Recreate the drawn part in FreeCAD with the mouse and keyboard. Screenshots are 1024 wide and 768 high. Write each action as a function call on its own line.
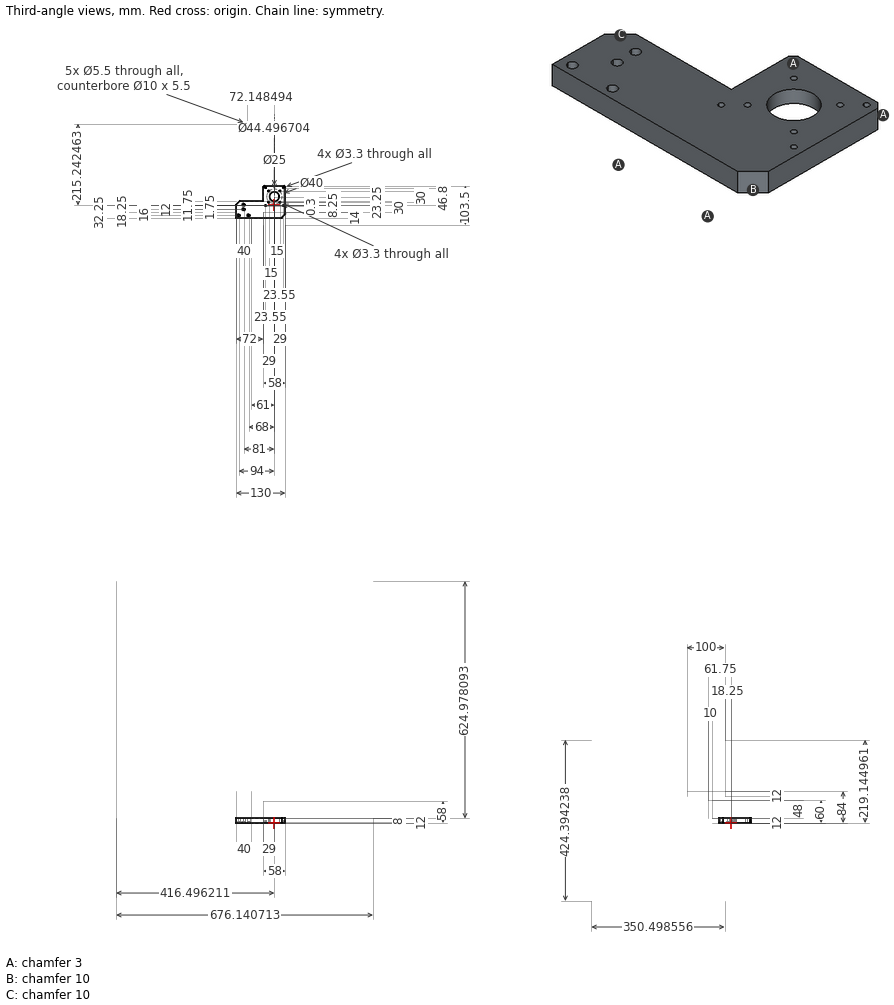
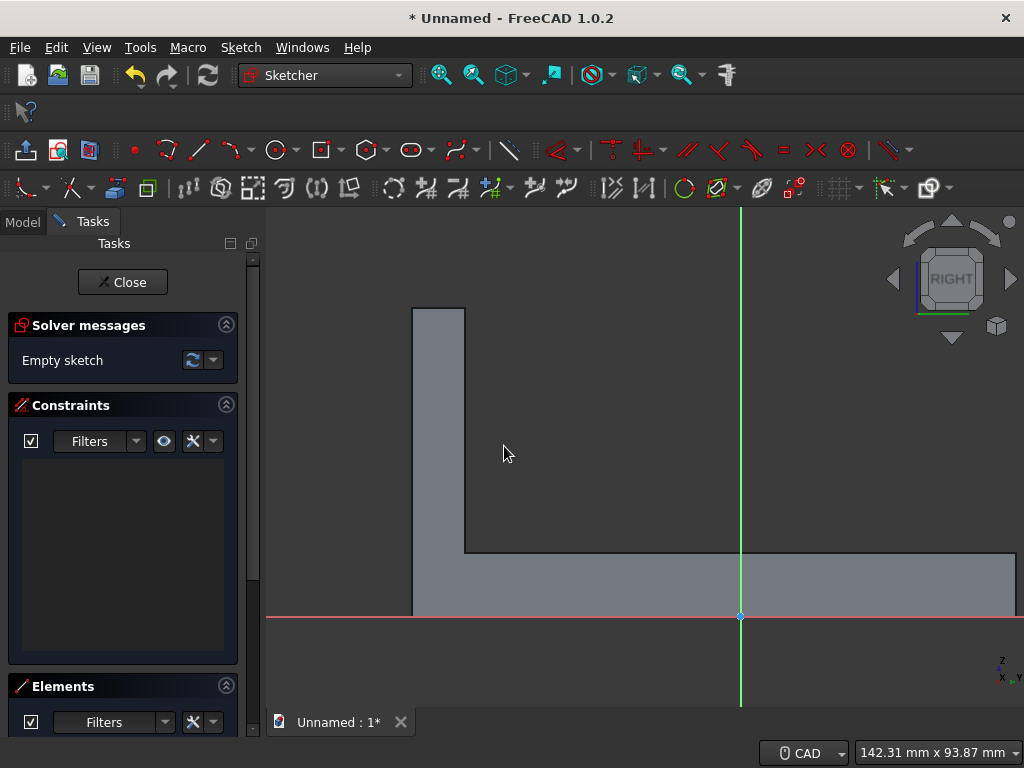
click(344, 150)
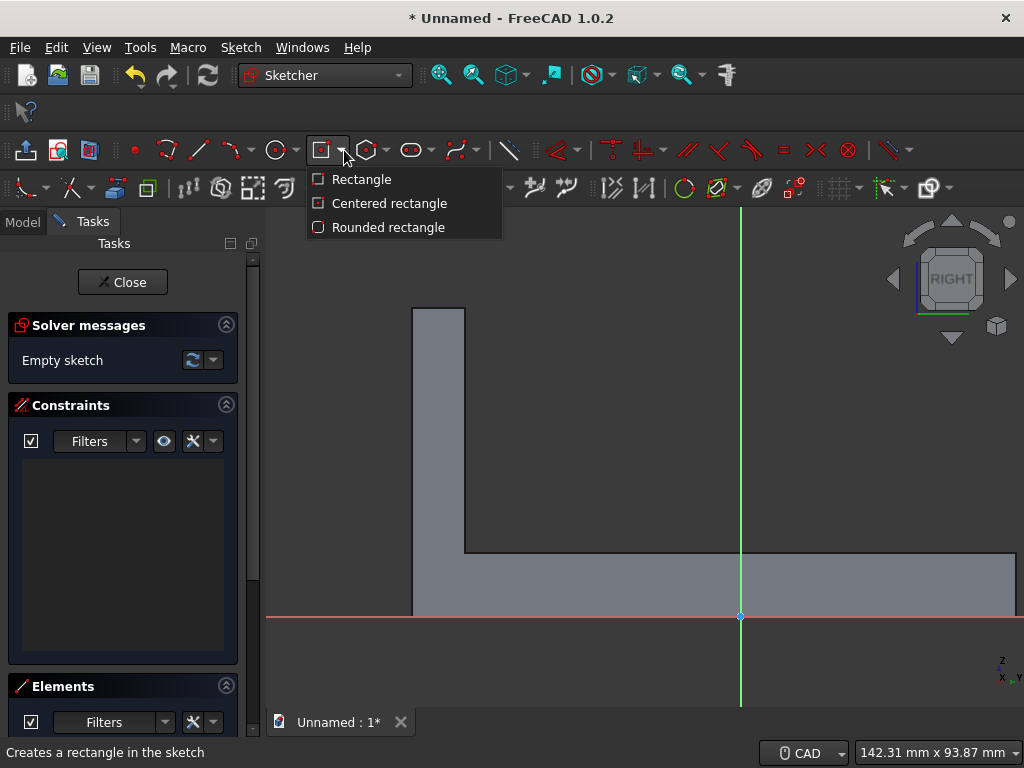
click(404, 179)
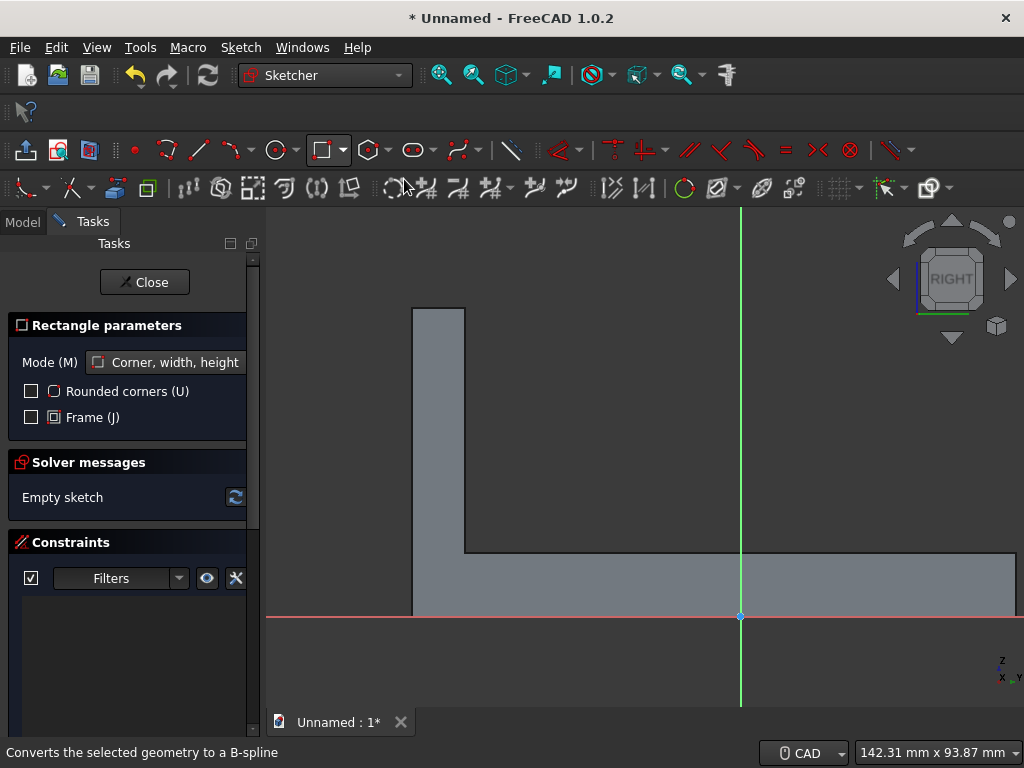
click(412, 297)
move(465, 553)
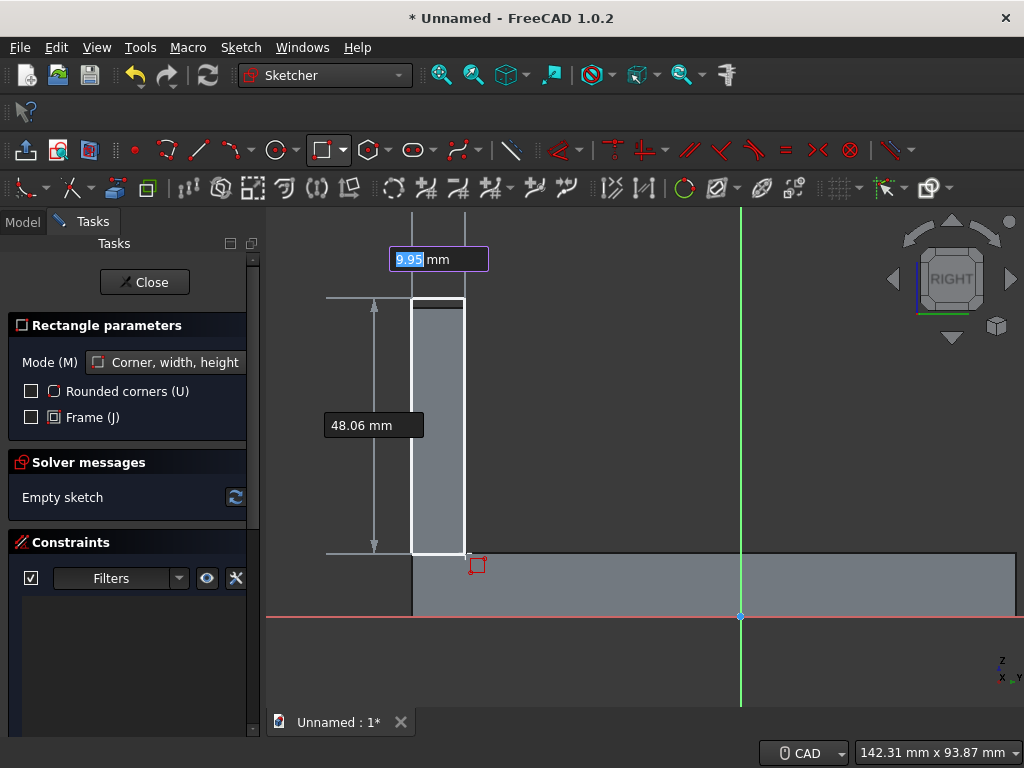
text(10)
key(Tab)
text(48)
key(Return)
key(Escape)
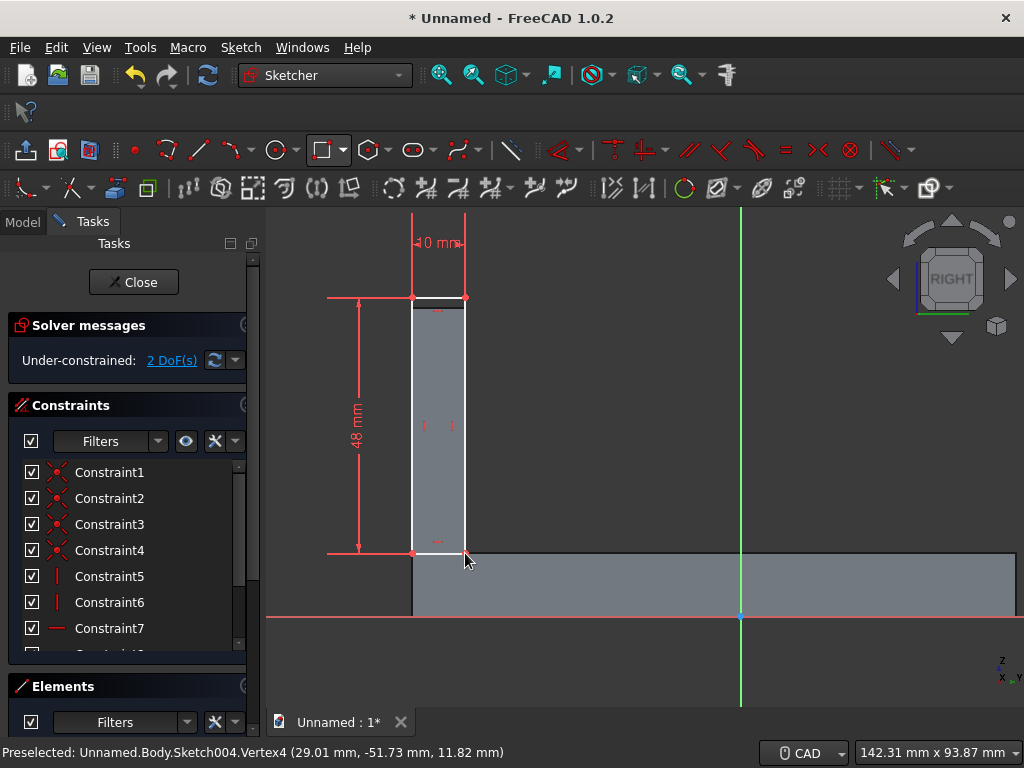
click(558, 150)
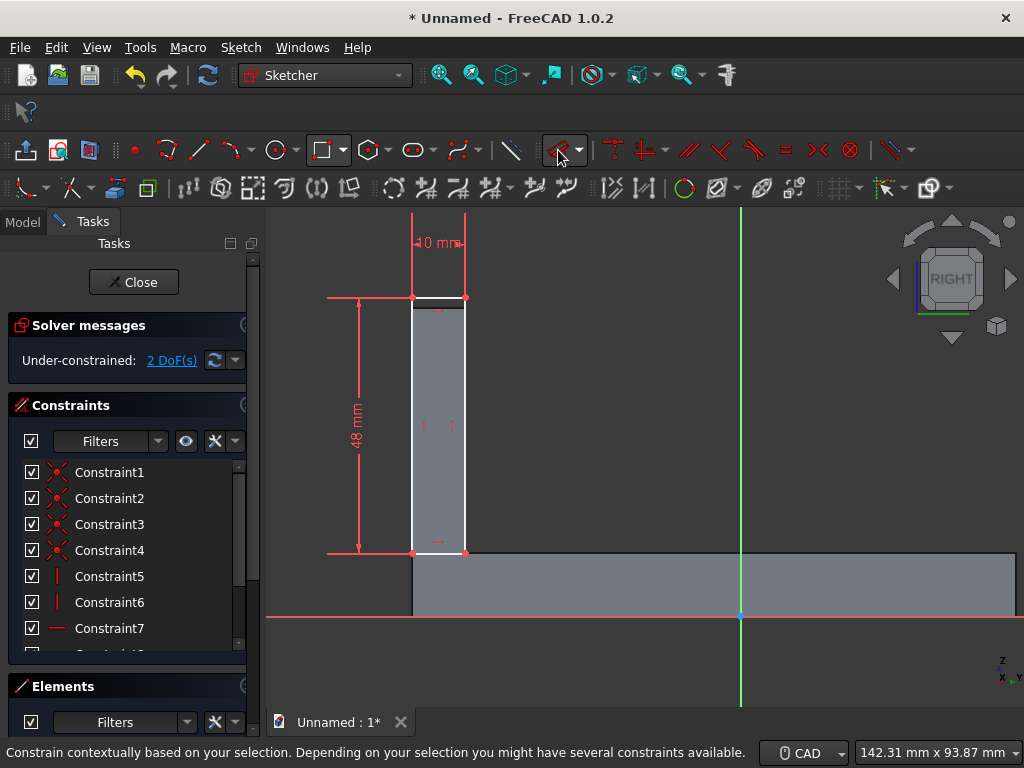
click(412, 298)
click(775, 457)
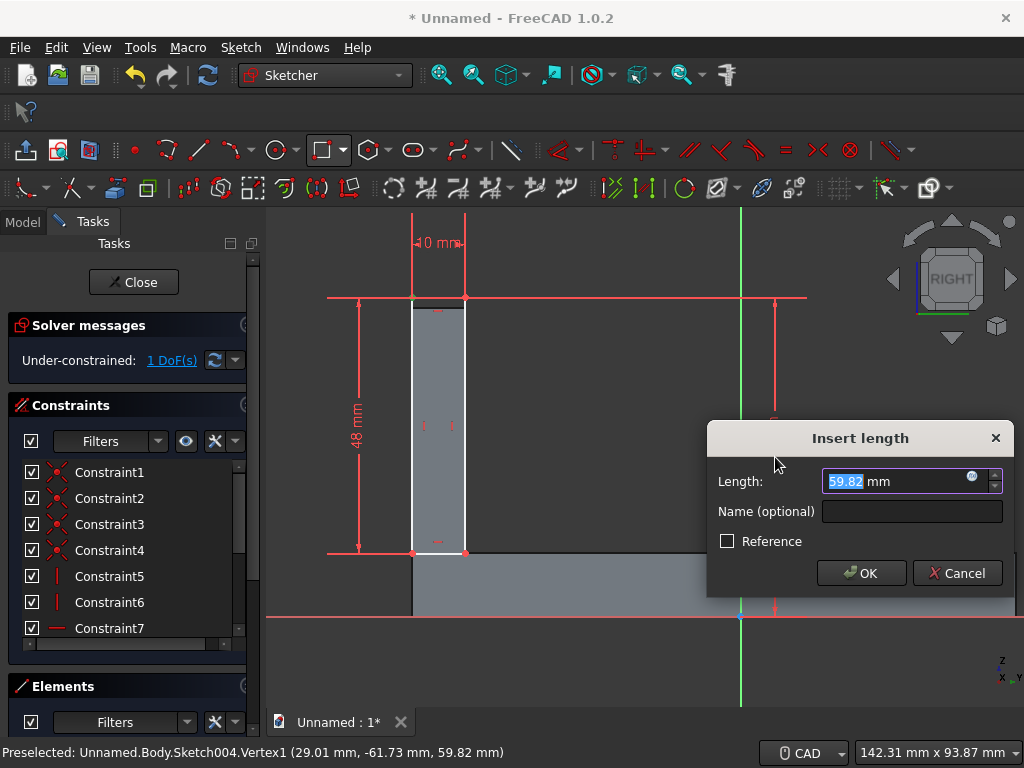
text(60)
key(Return)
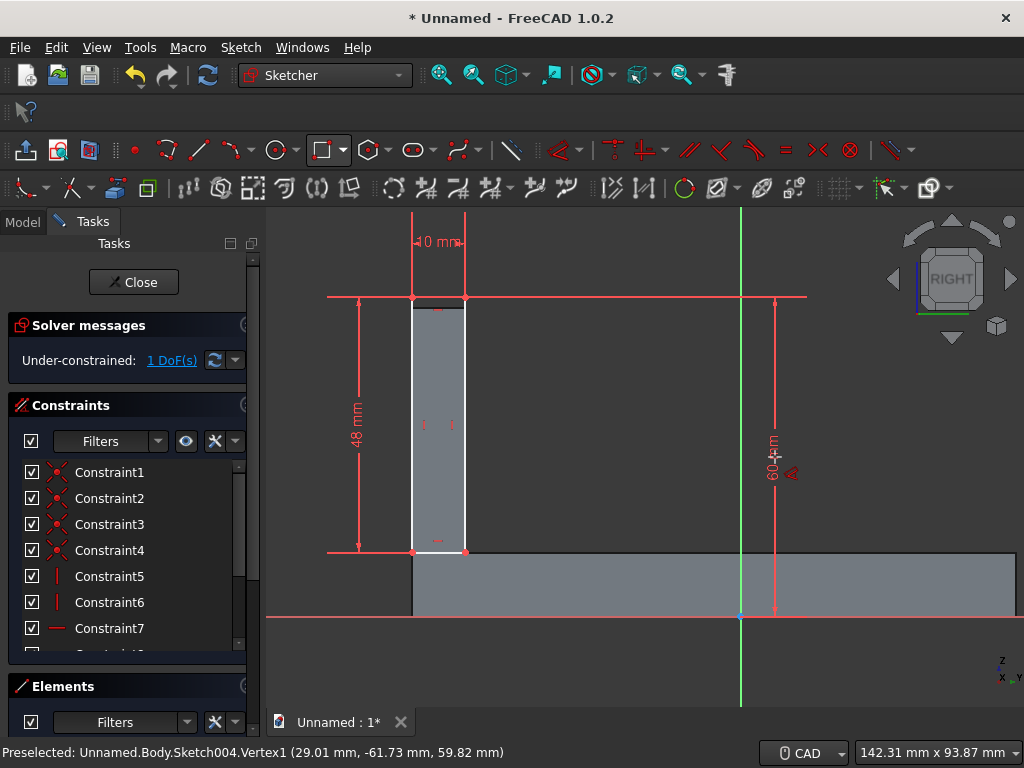
click(412, 297)
click(576, 651)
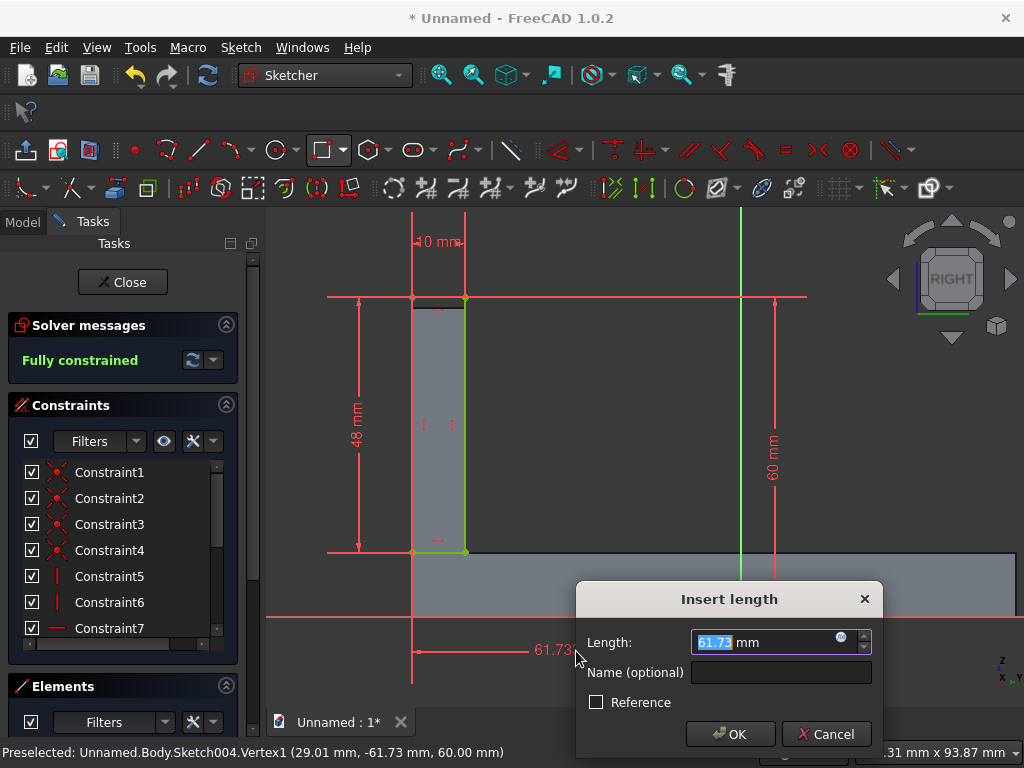
text(61.75)
key(Return)
key(Escape)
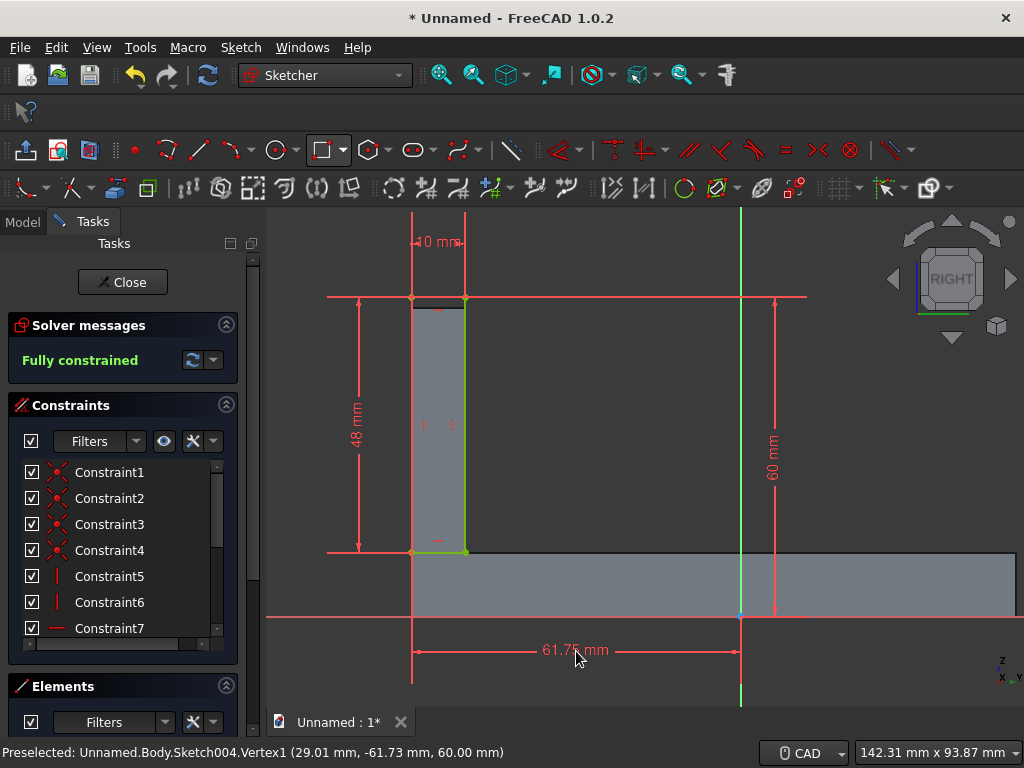
click(123, 282)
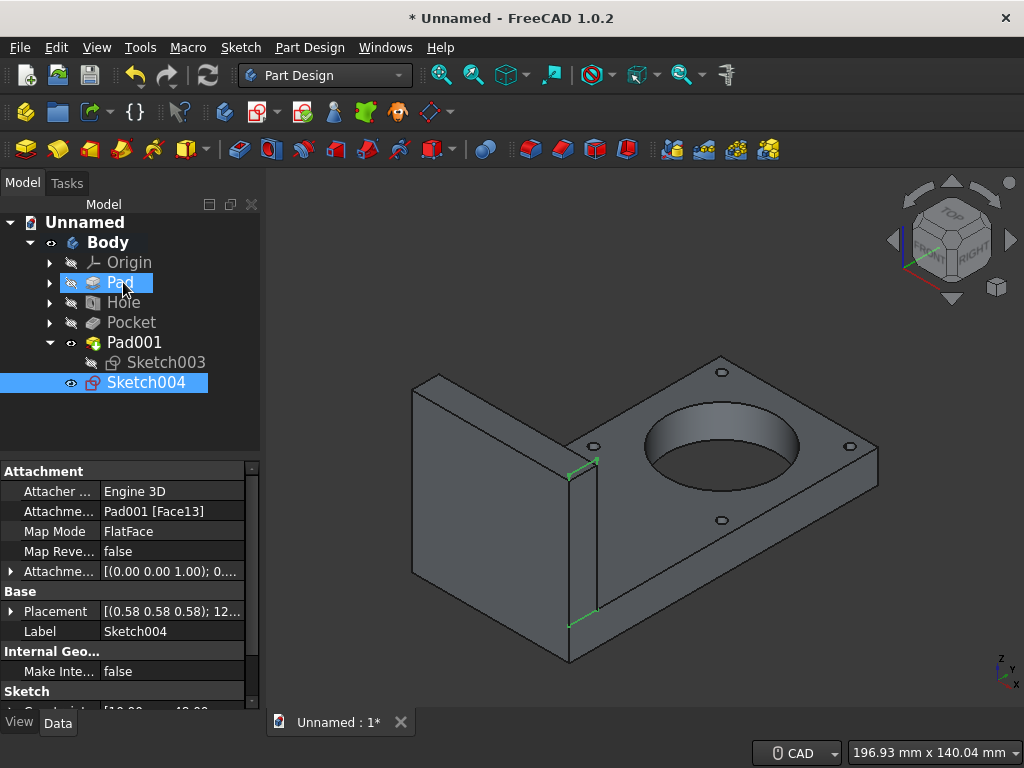
click(240, 150)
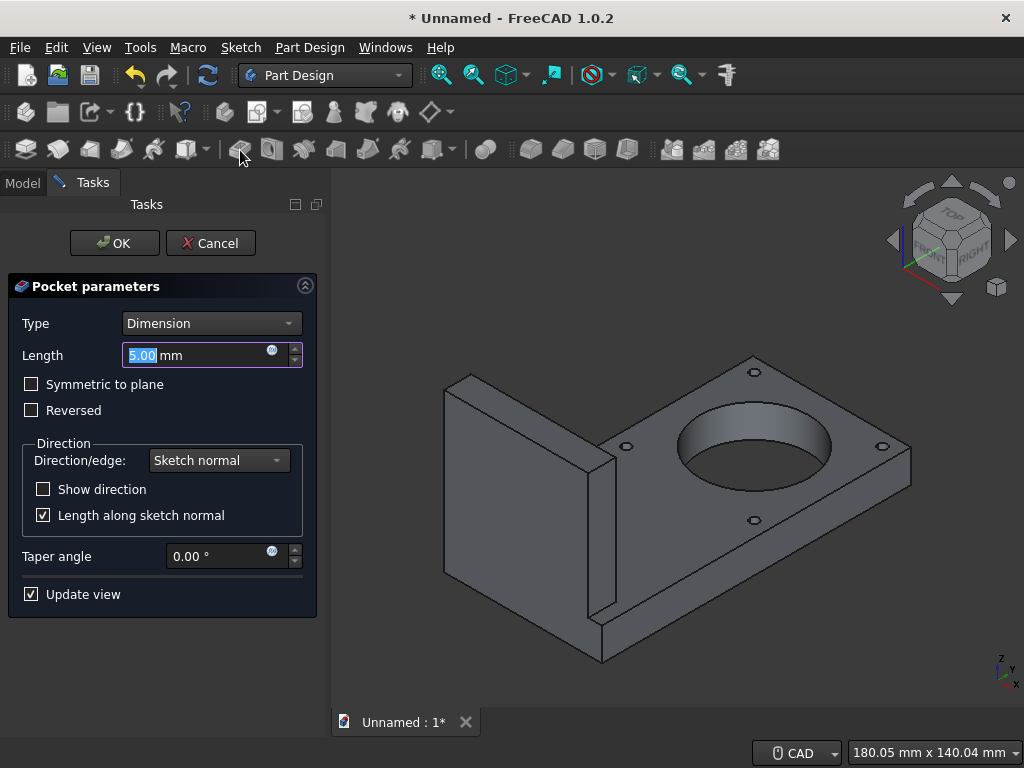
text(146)
key(Tab)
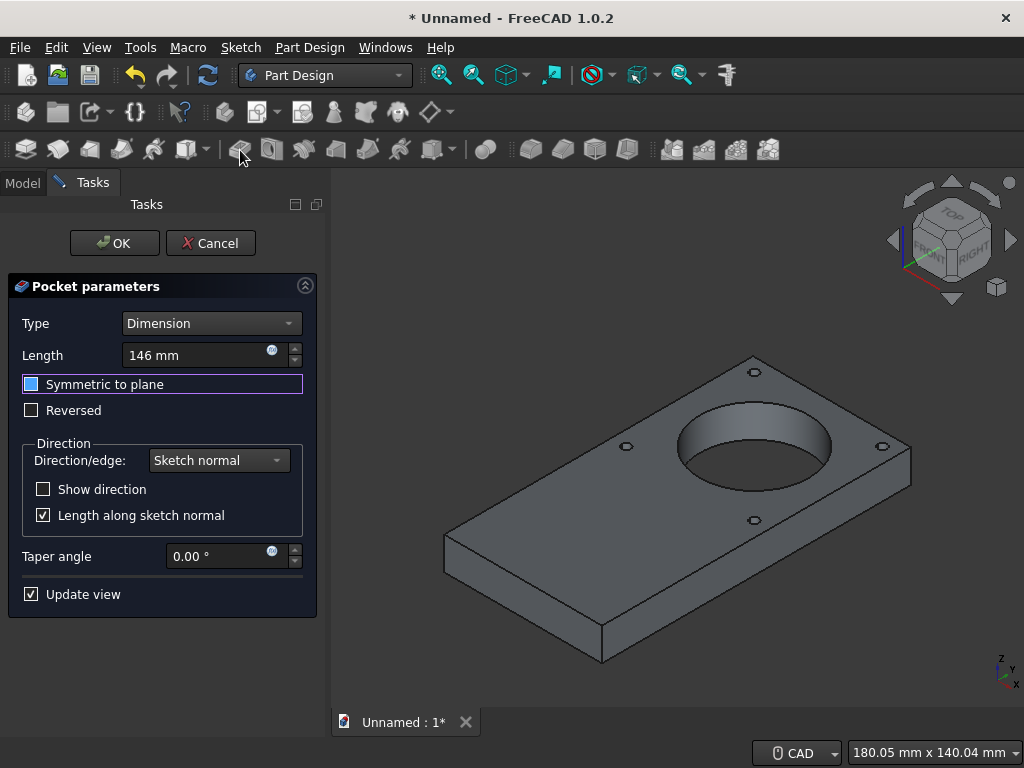
click(115, 243)